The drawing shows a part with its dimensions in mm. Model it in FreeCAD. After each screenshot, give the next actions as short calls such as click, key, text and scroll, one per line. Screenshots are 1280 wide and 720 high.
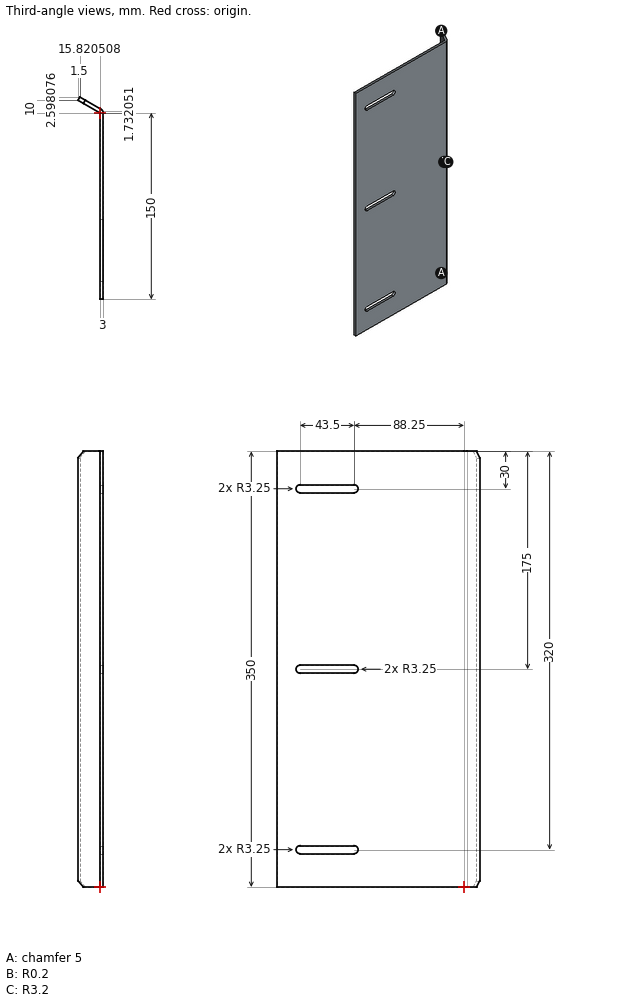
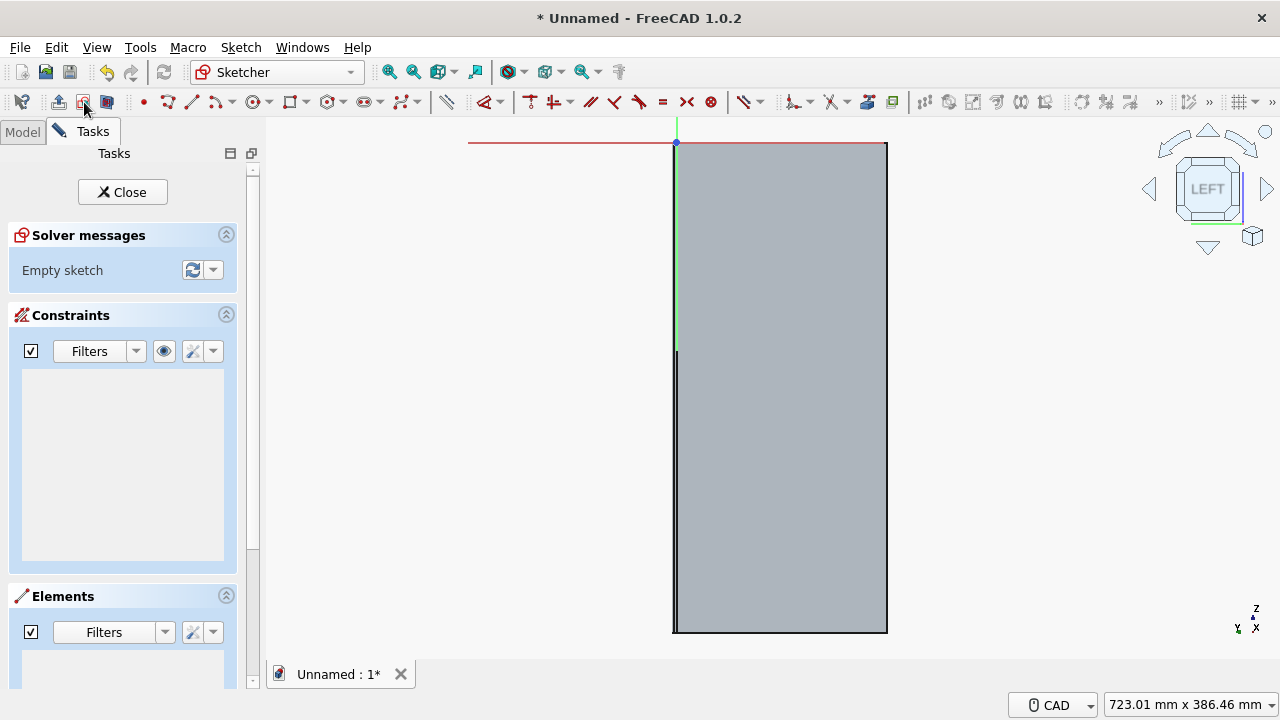
scroll(847, 159, up, 11)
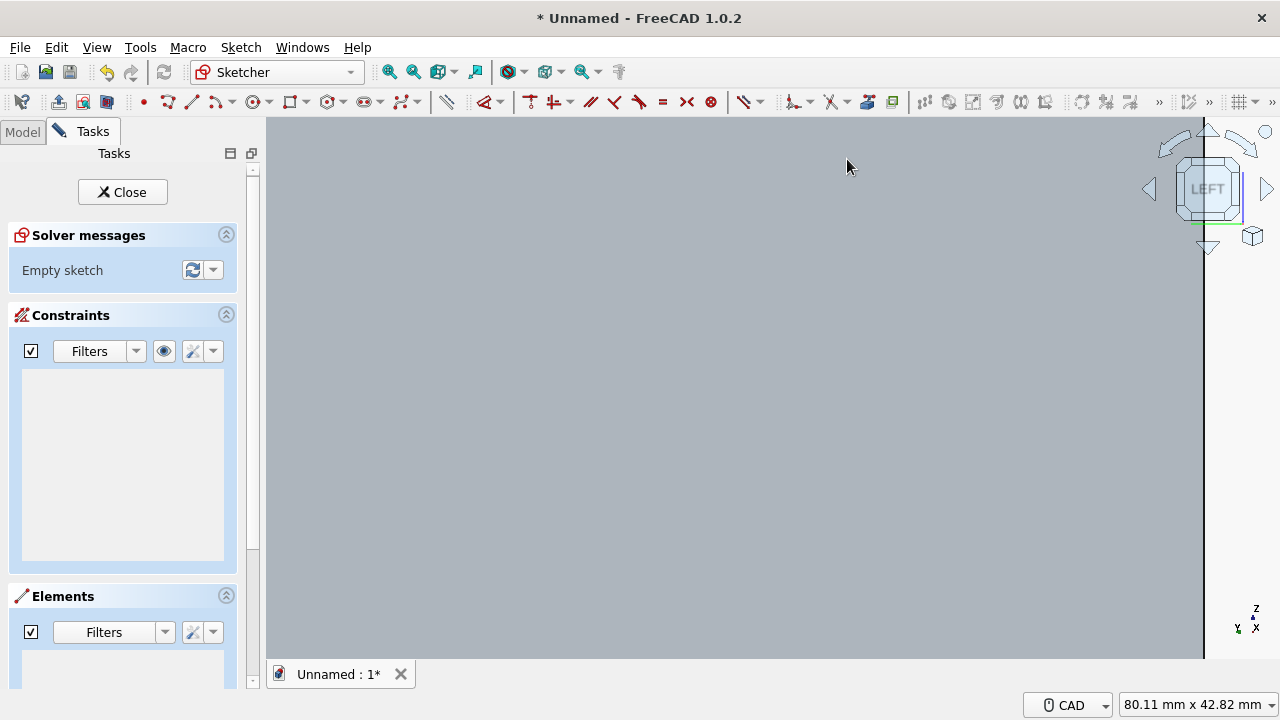
click(364, 102)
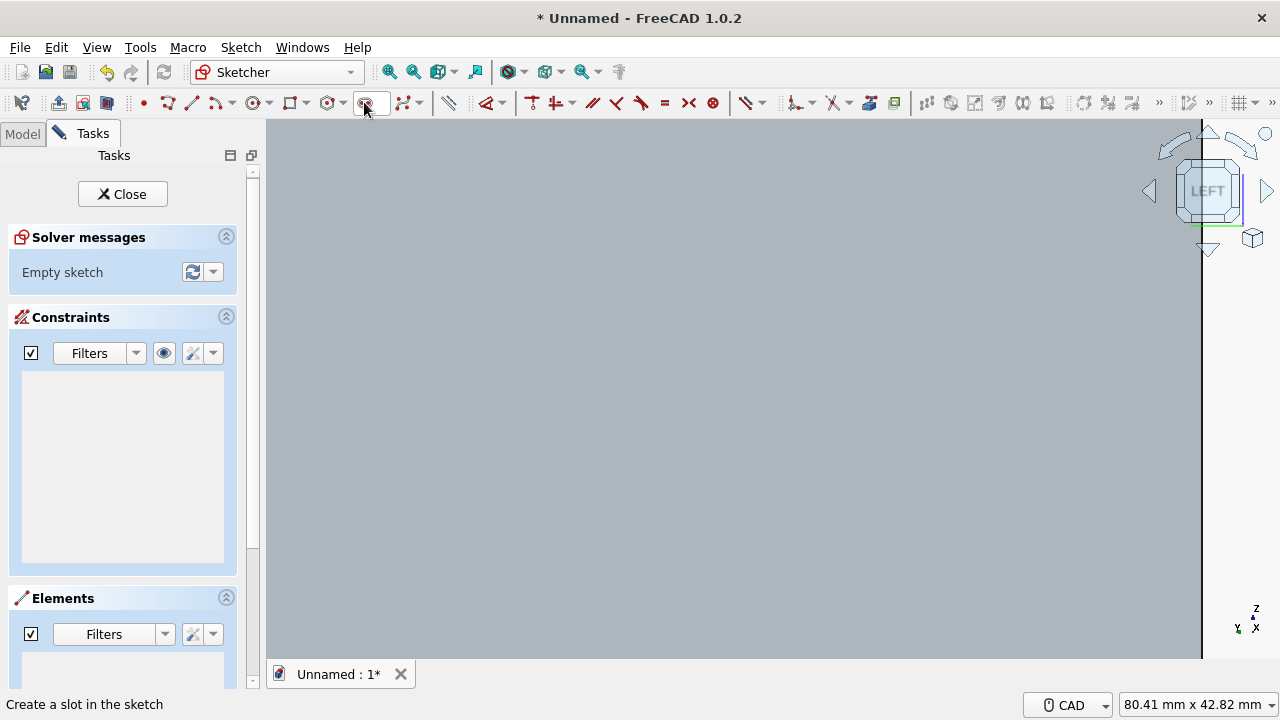
click(423, 391)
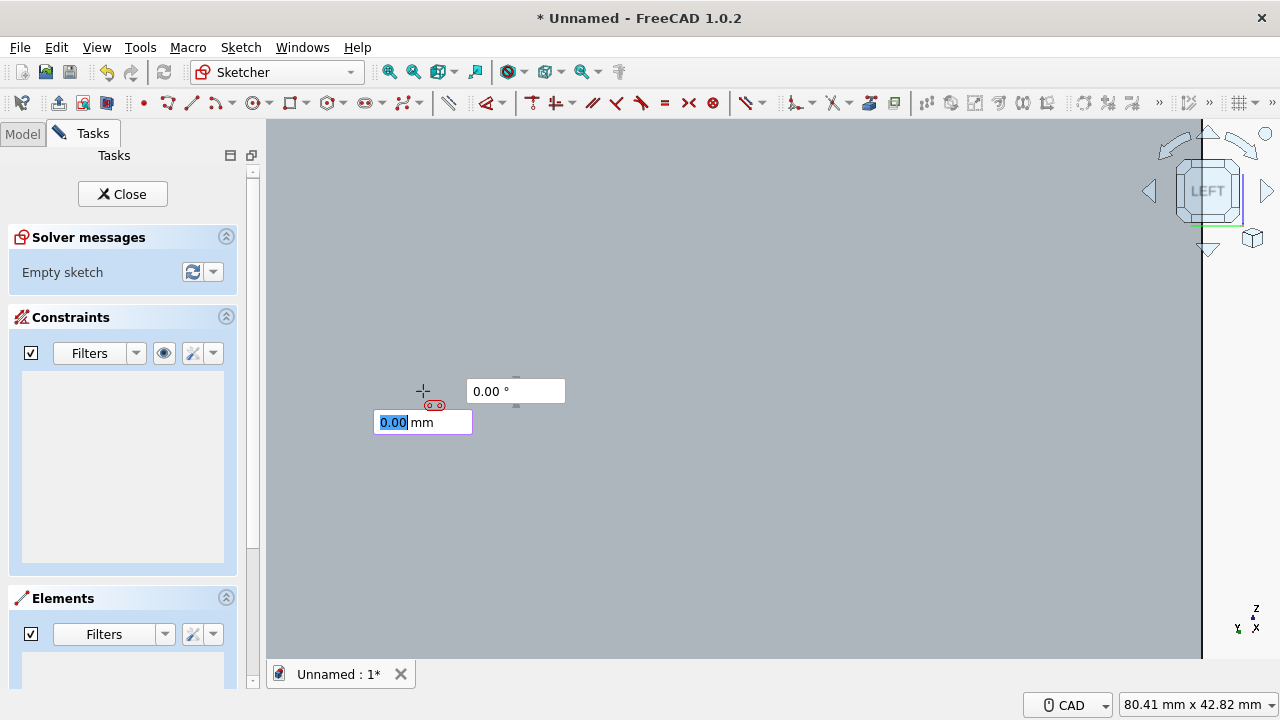
click(972, 391)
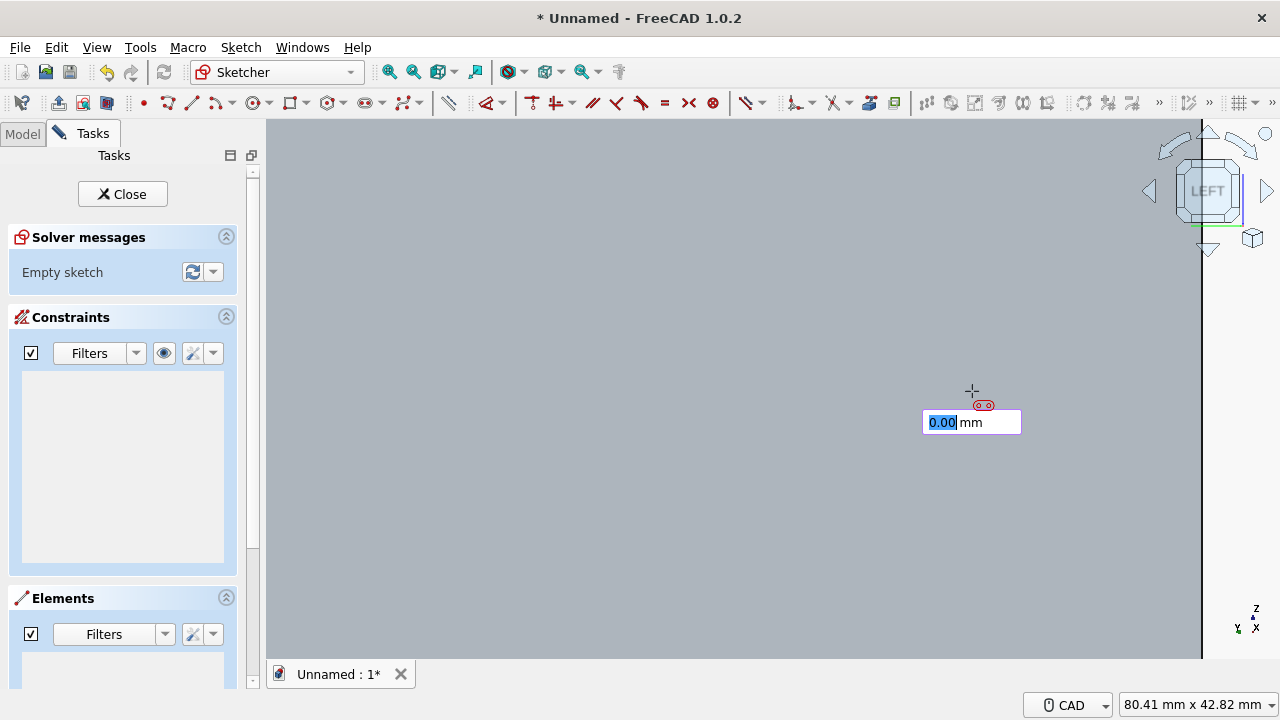
click(698, 432)
key(Escape)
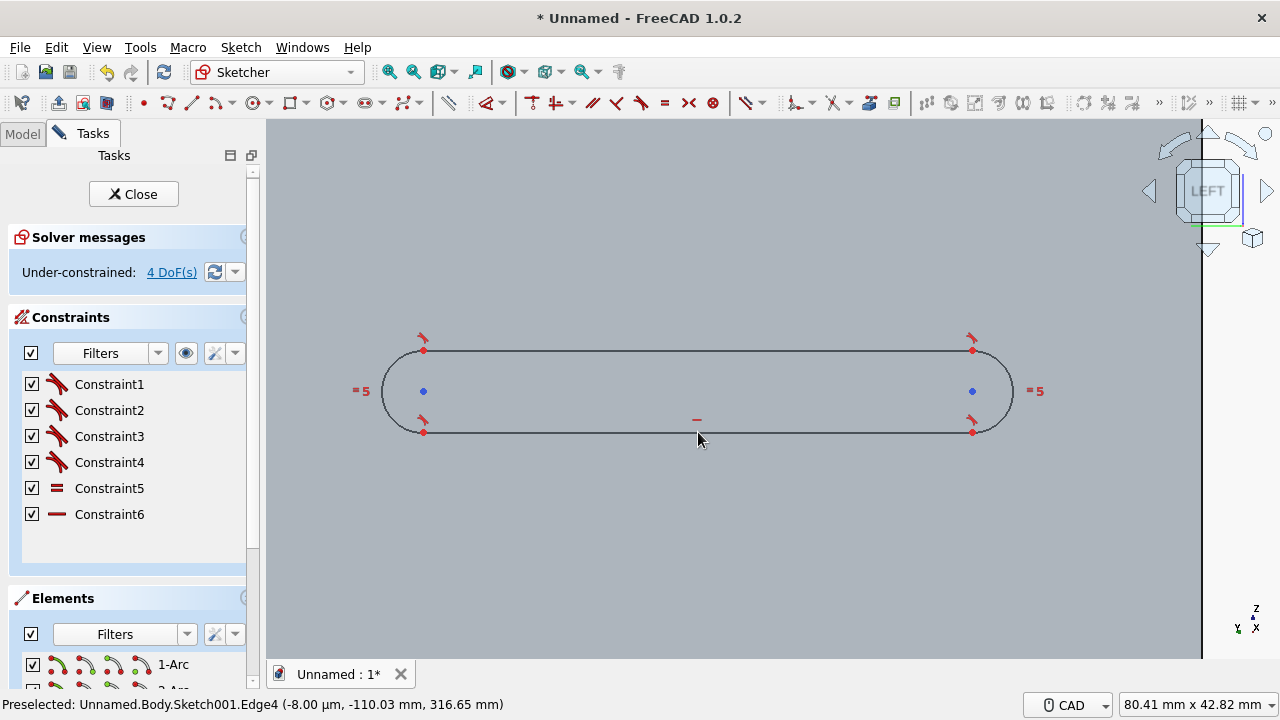
key(d)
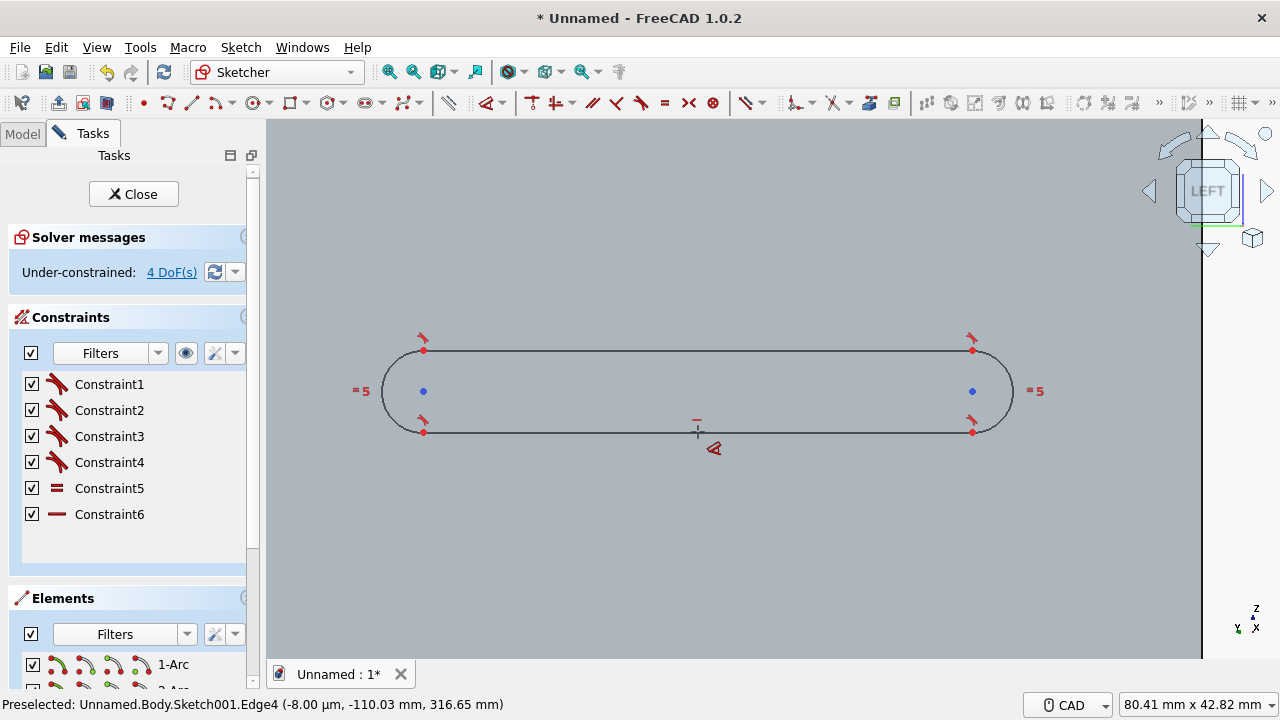
click(390, 368)
click(364, 349)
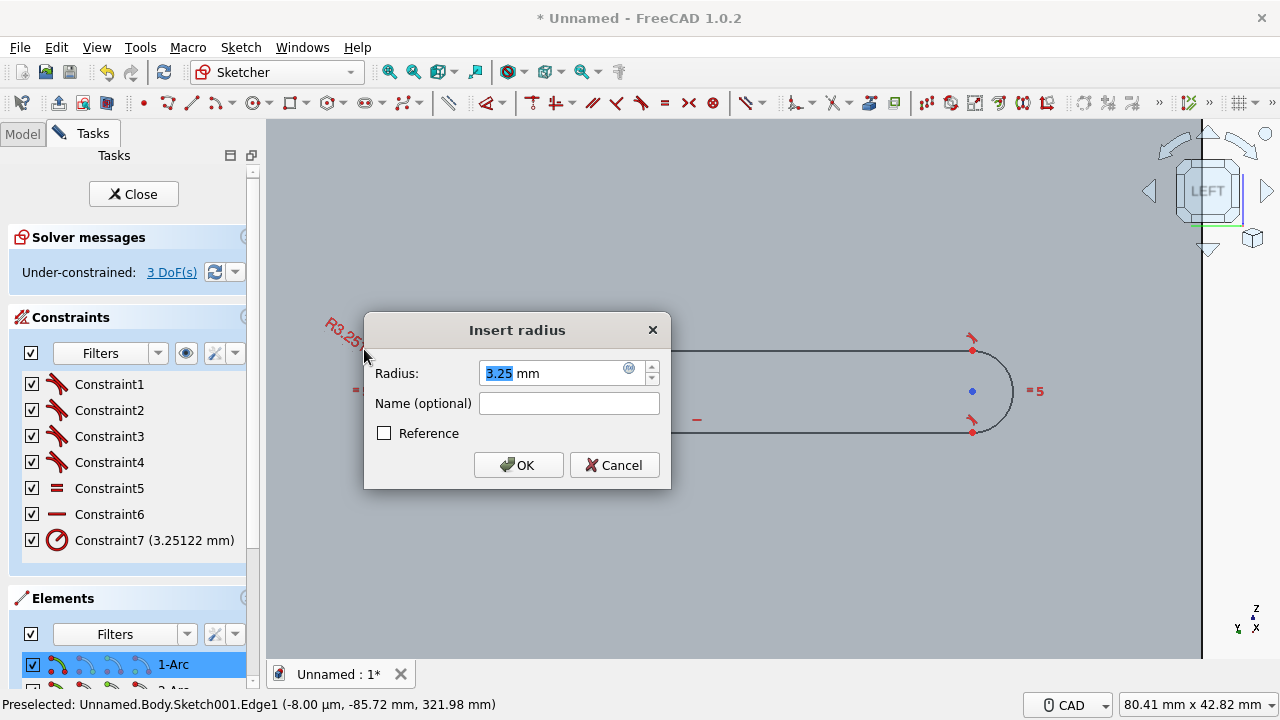
text(3.25)
key(Return)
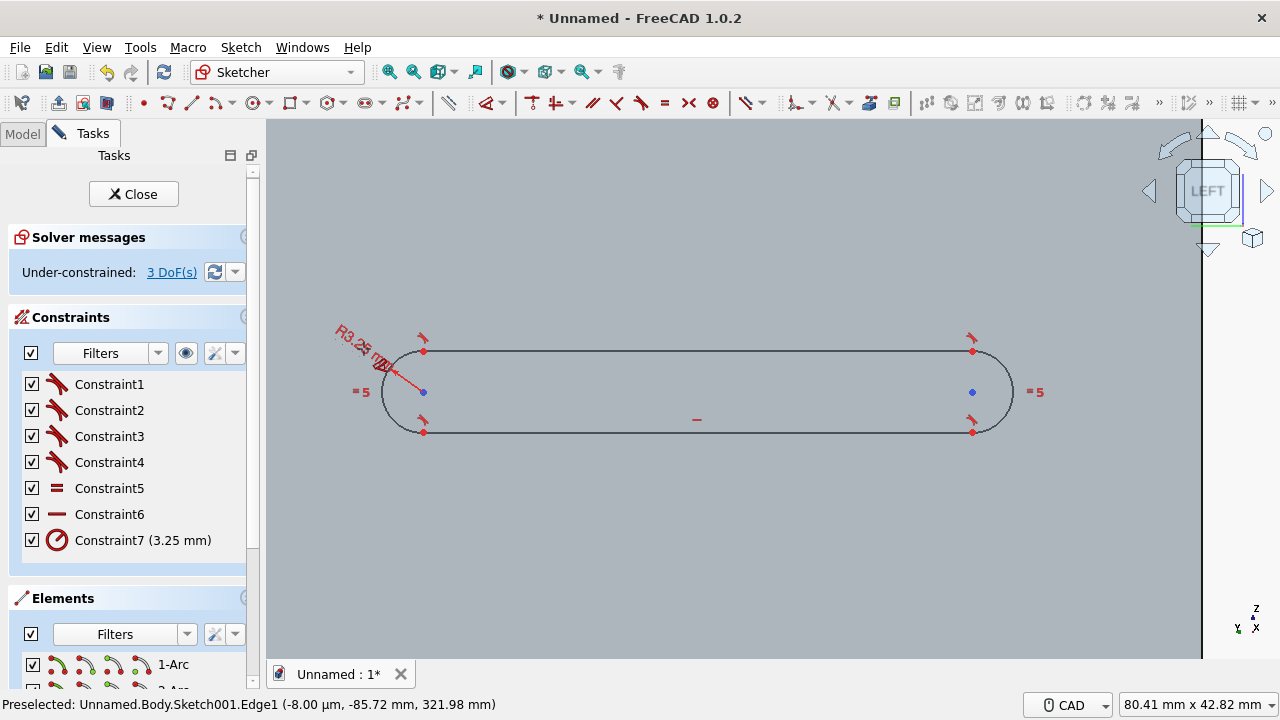
click(423, 392)
click(457, 270)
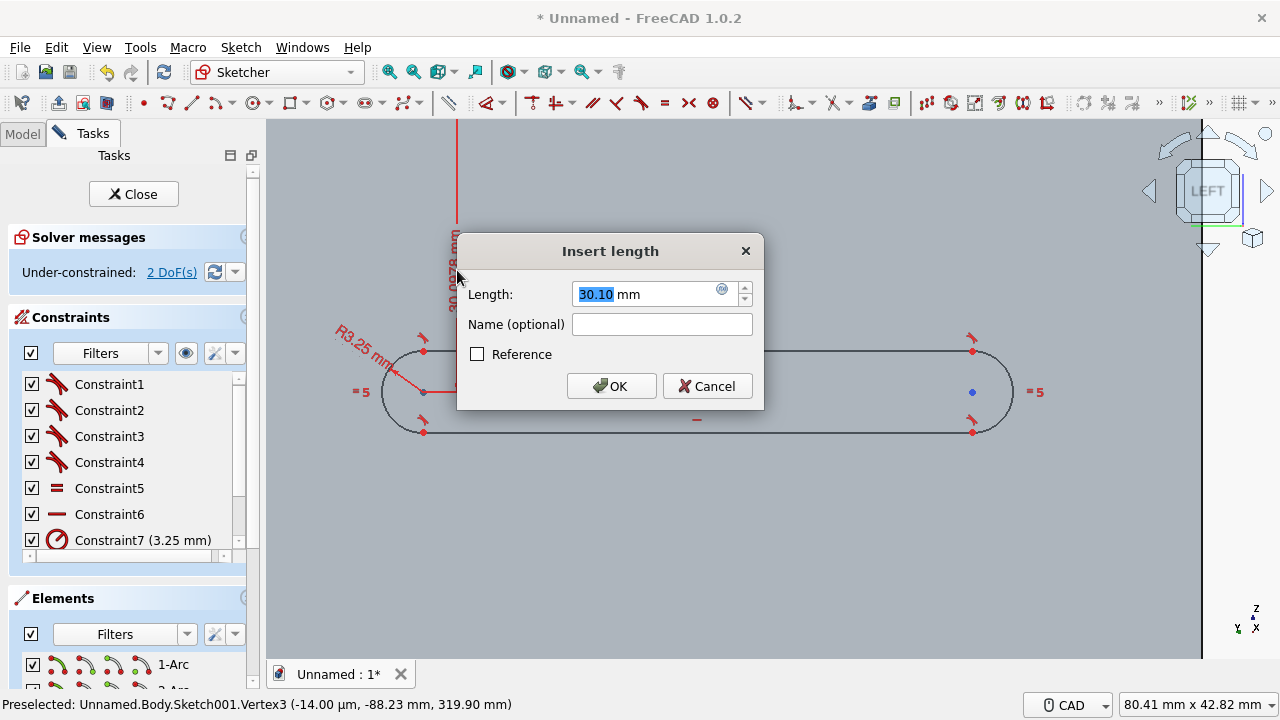
text(30)
key(Return)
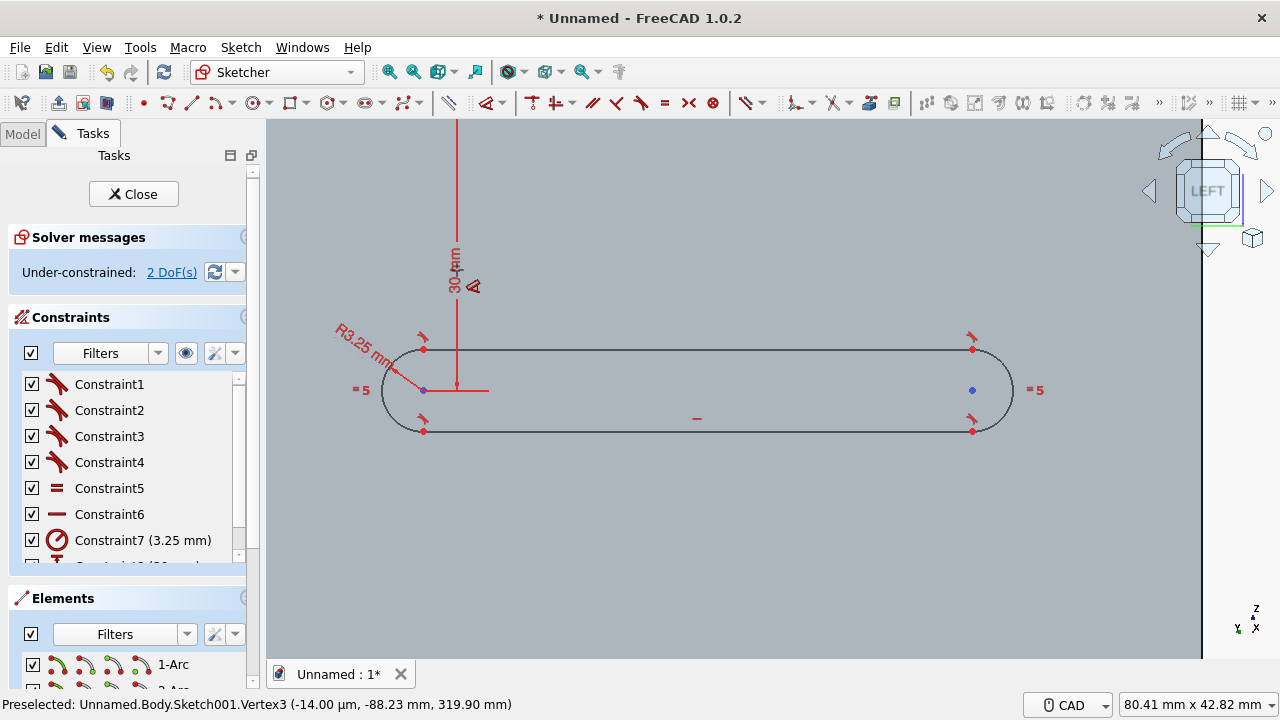
click(588, 350)
click(698, 316)